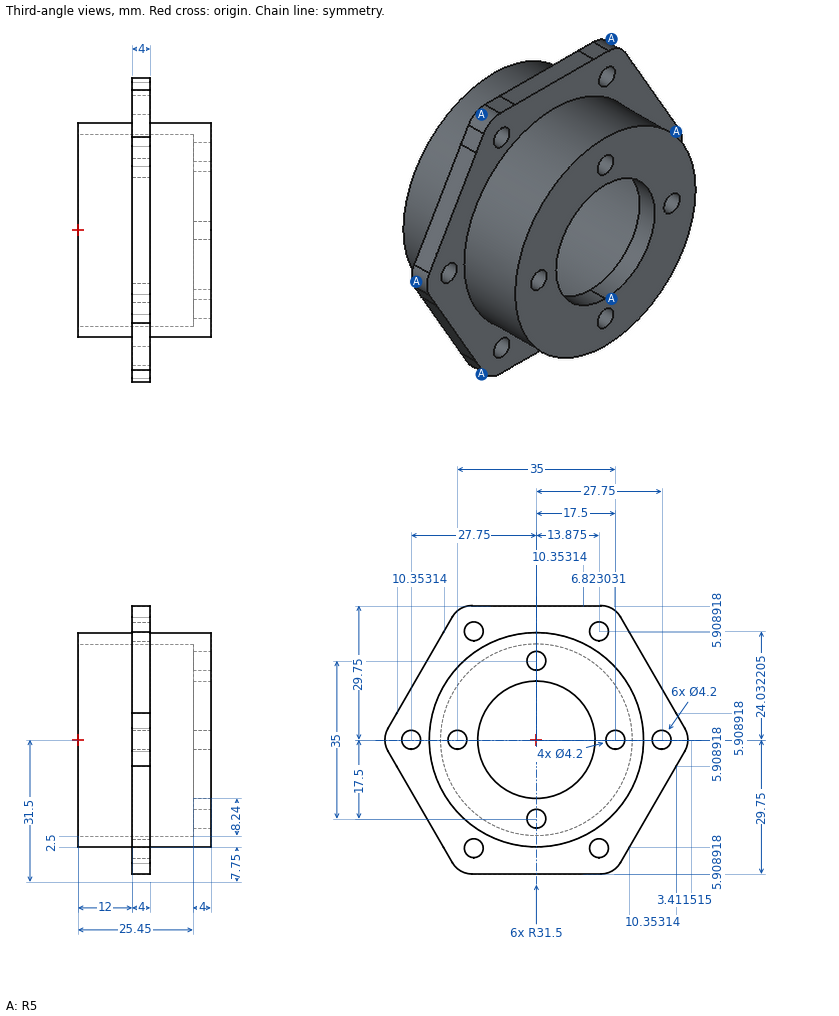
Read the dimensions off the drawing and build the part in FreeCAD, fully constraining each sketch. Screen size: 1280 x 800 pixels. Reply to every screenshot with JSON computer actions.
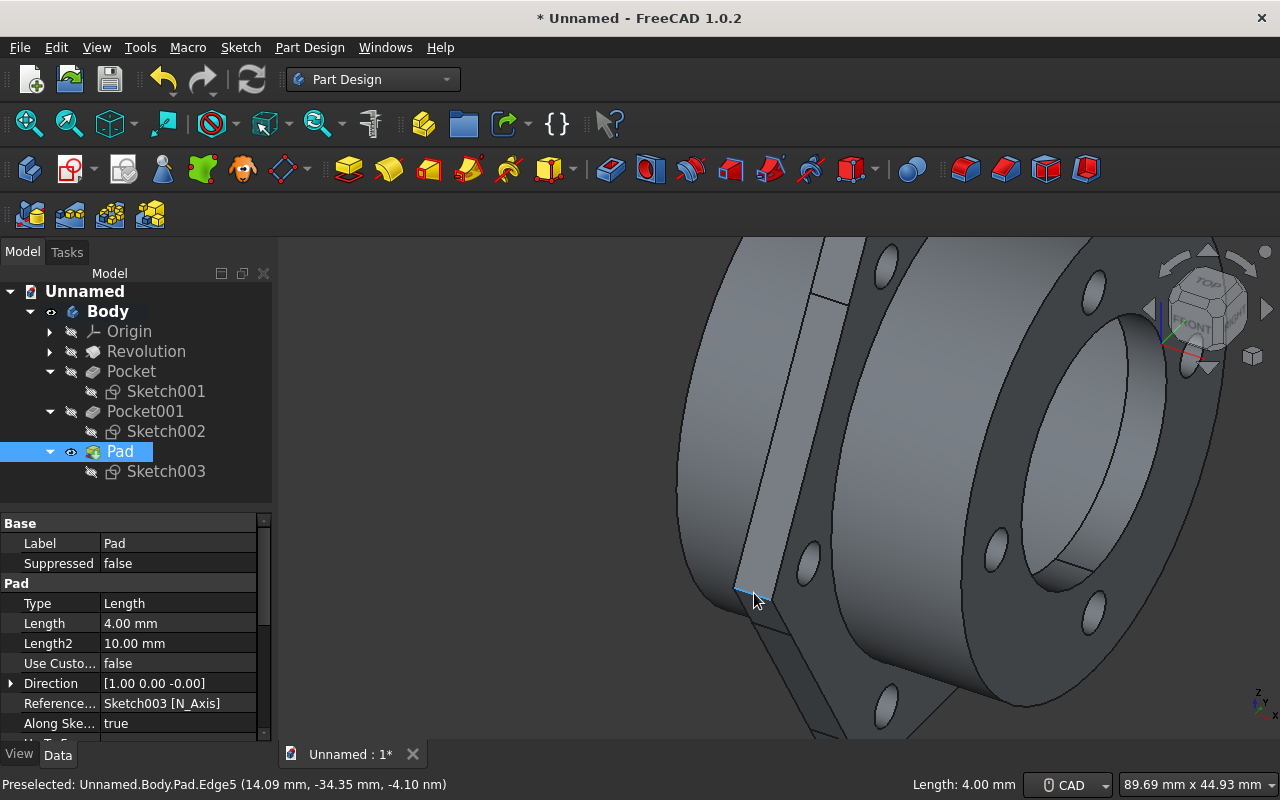
{"action": "key", "text": "v f"}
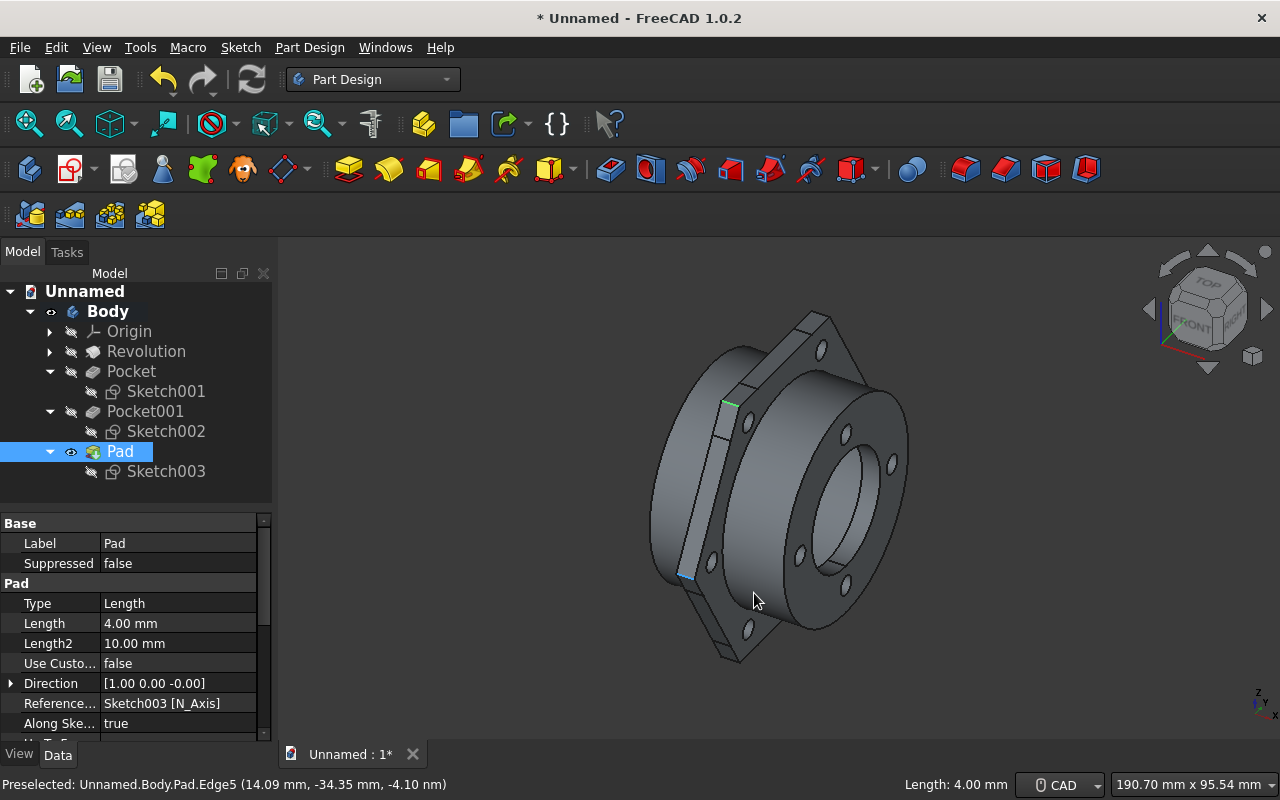
{"action": "key", "text": "0"}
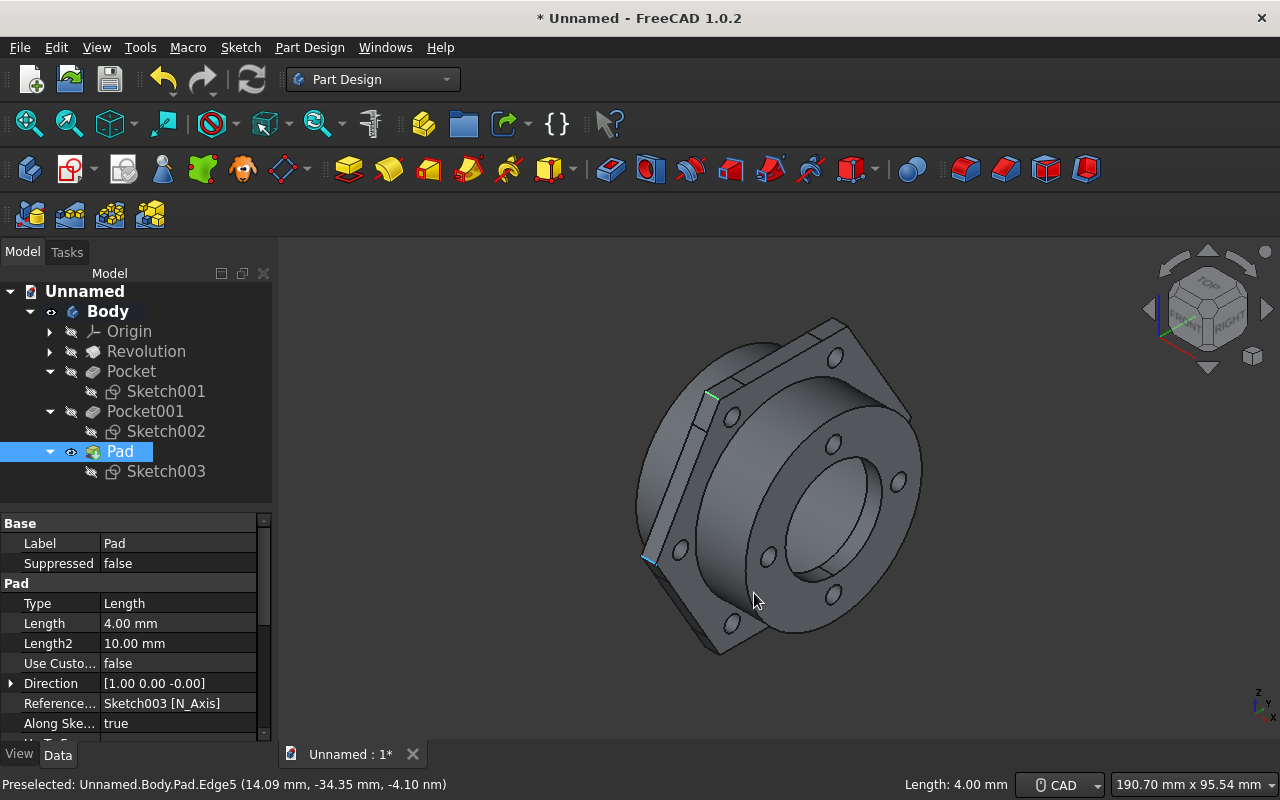
{"action": "scroll", "coordinate": [649, 559], "scroll_direction": "up", "scroll_amount": 4}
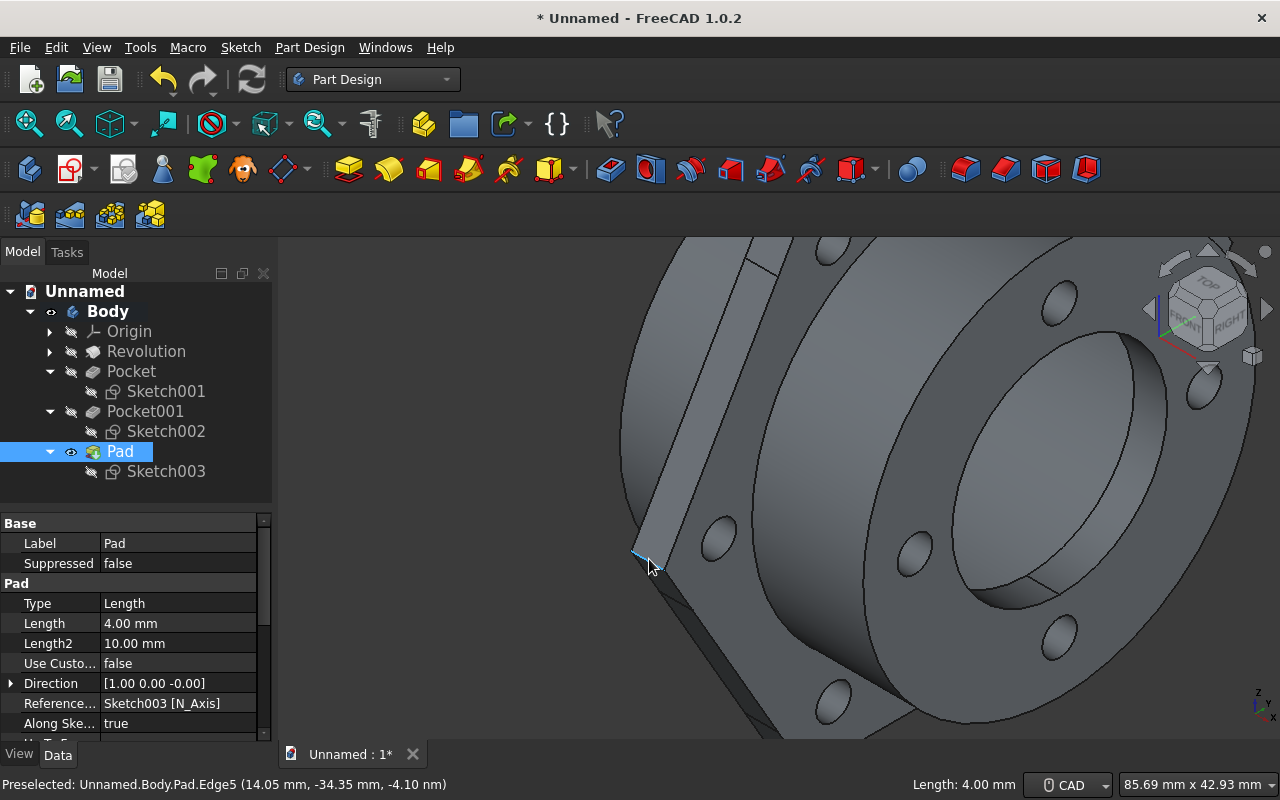
{"action": "key", "text": "v f"}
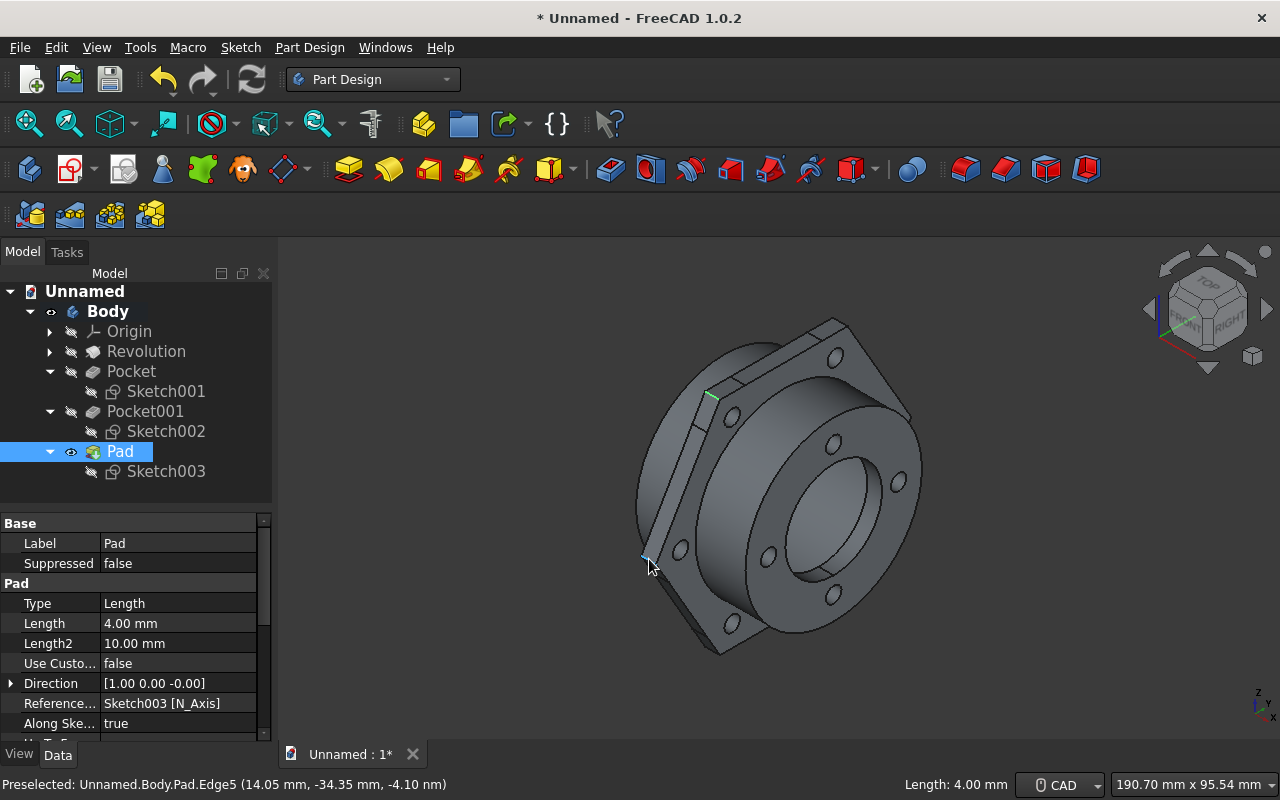
{"action": "key", "text": "2"}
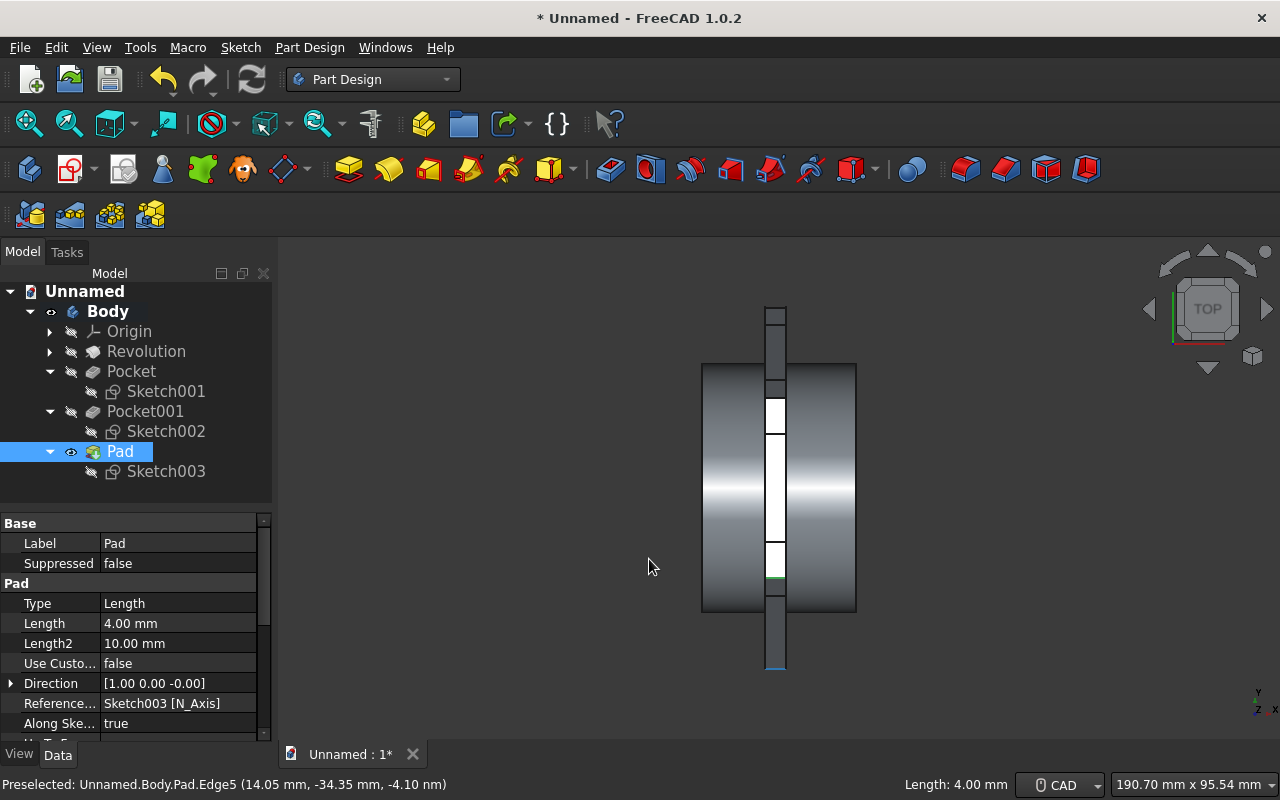
{"action": "left_click", "coordinate": [775, 397], "text": "ctrl"}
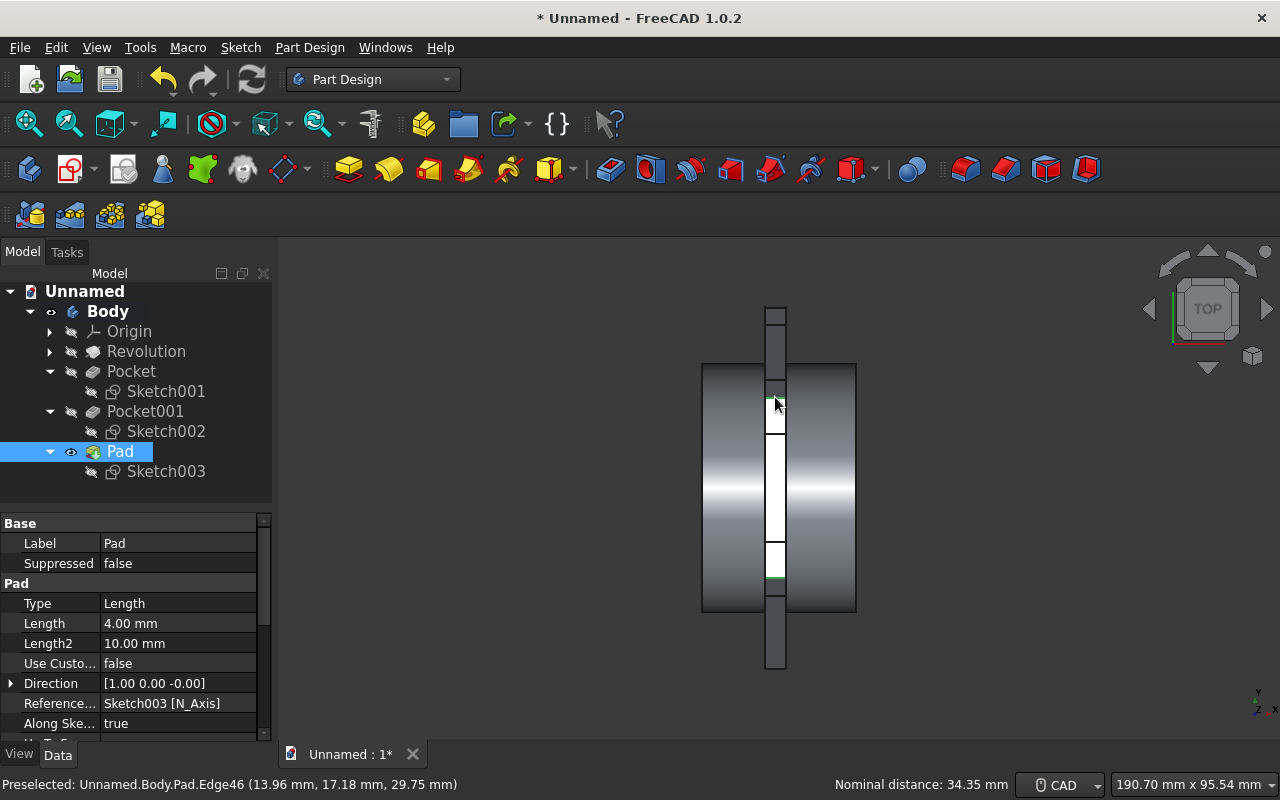
{"action": "scroll", "coordinate": [775, 667], "scroll_direction": "up", "scroll_amount": 4}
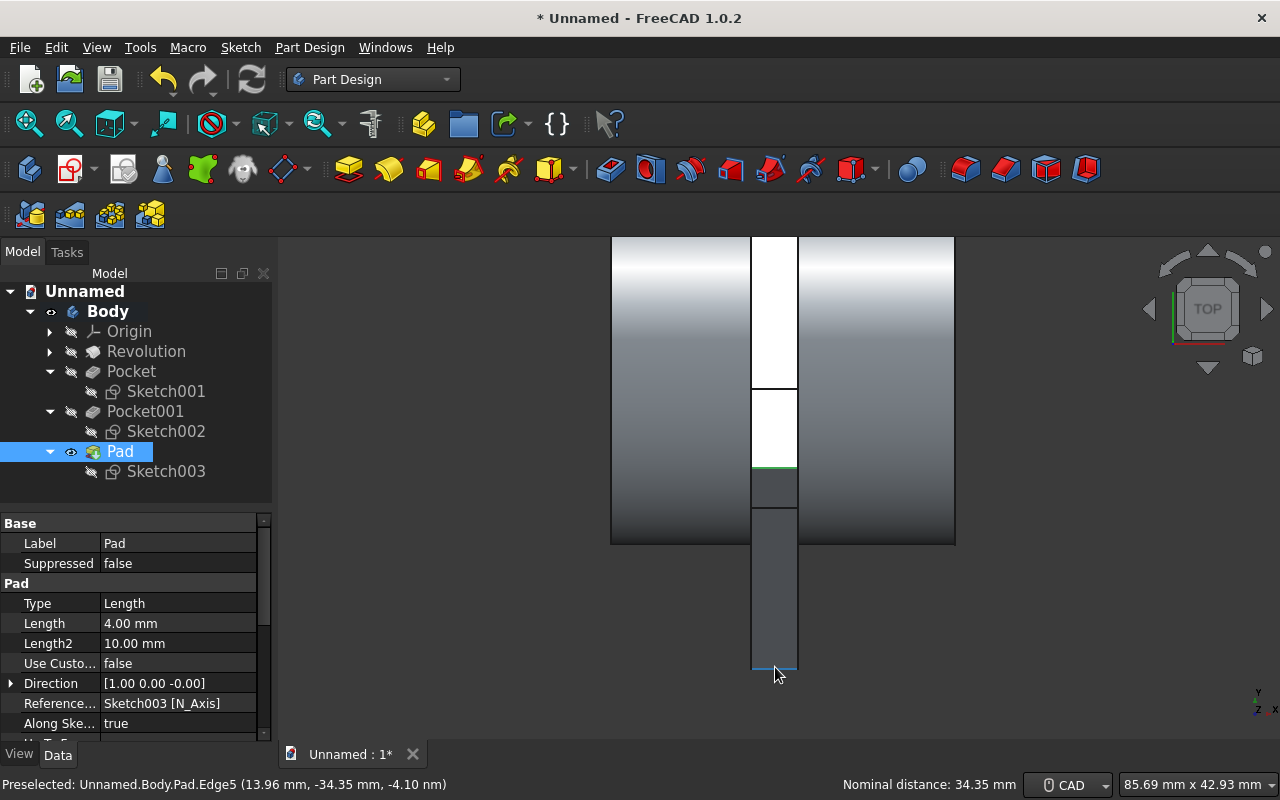
{"action": "key", "text": "v f"}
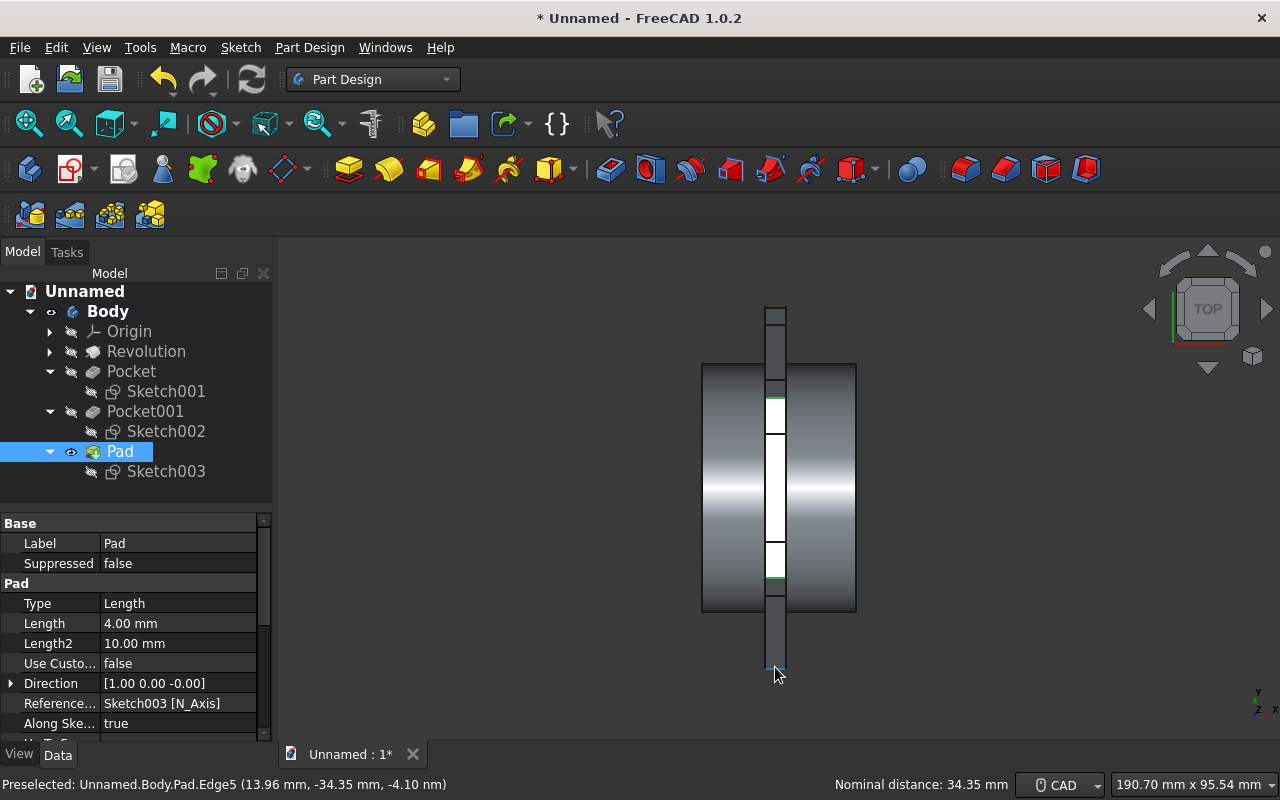
{"action": "key", "text": "1"}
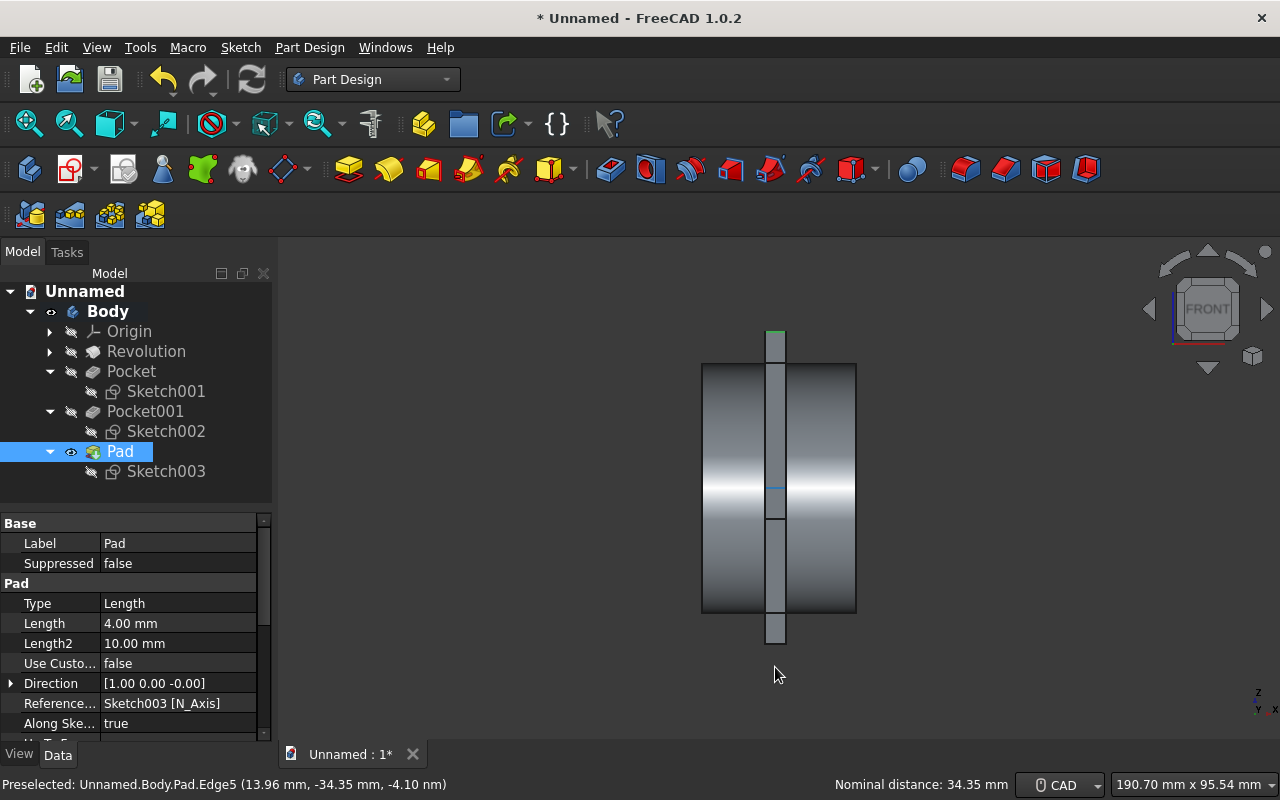
{"action": "left_click", "coordinate": [775, 487], "text": "ctrl"}